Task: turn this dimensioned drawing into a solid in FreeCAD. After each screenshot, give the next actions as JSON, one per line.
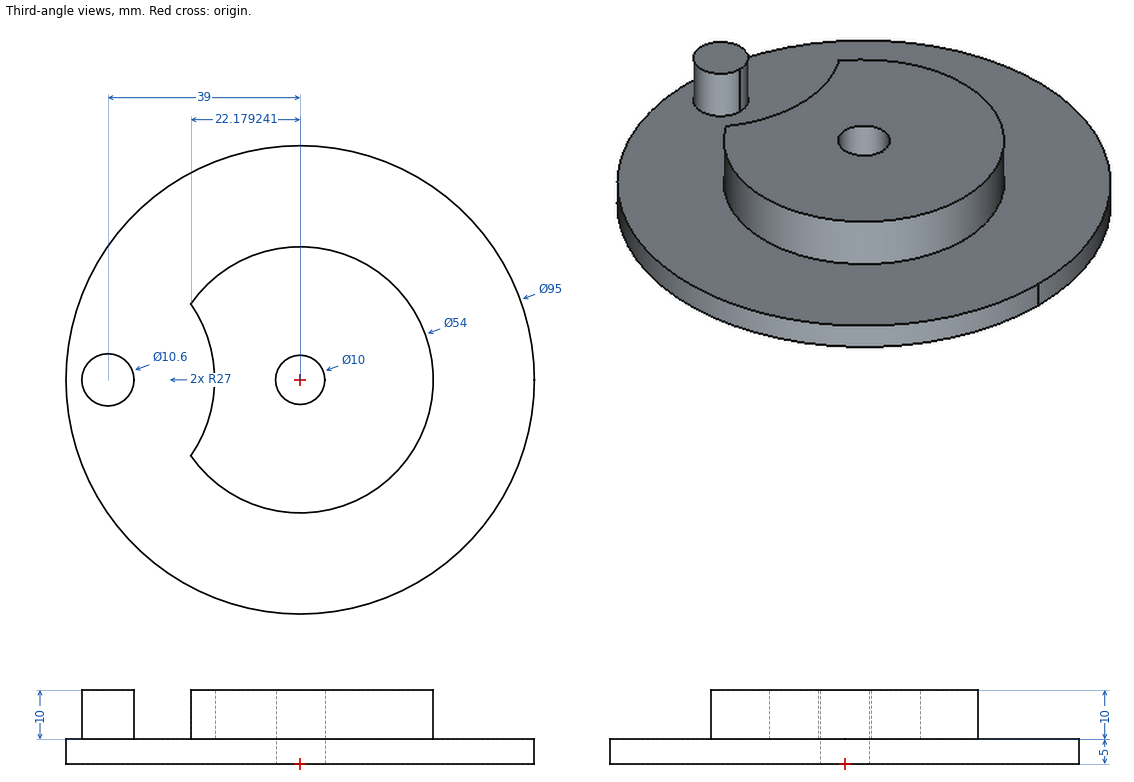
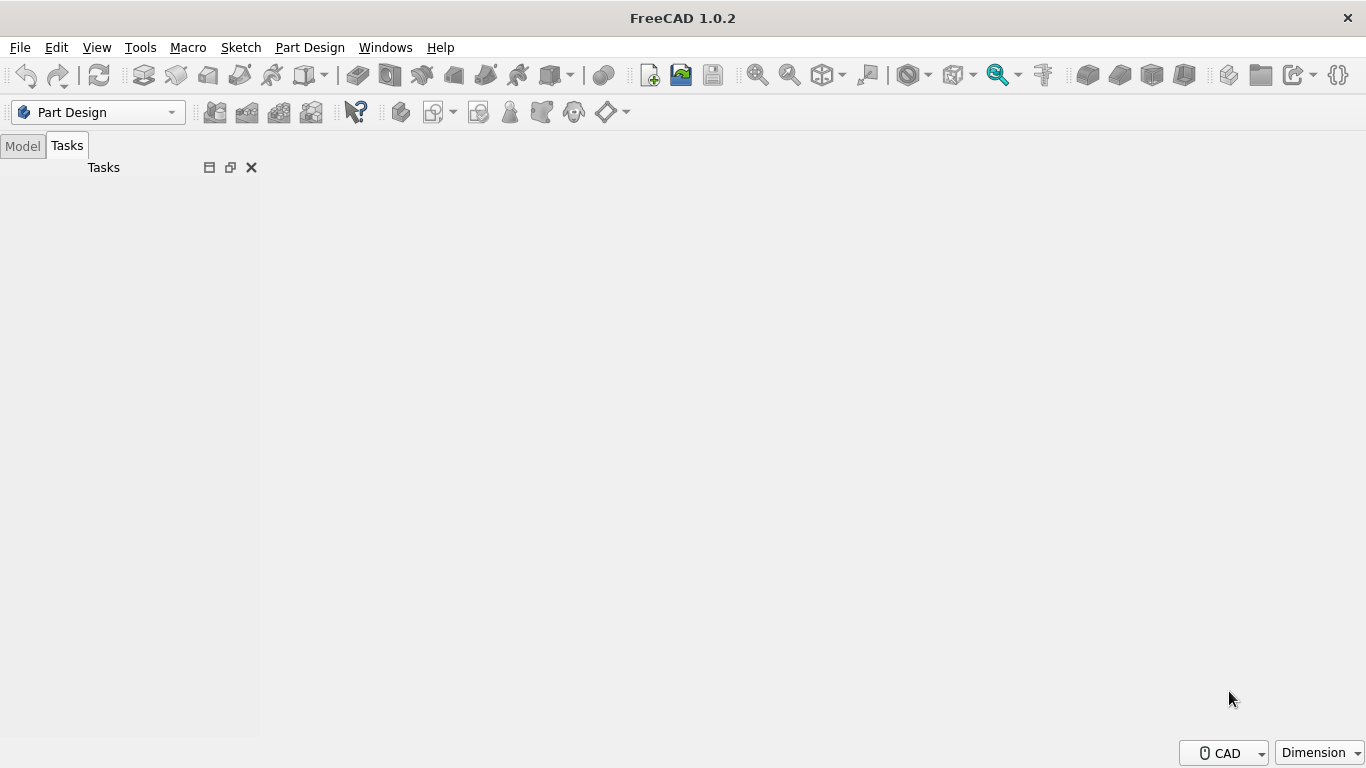
{"action": "key", "text": "ctrl+n"}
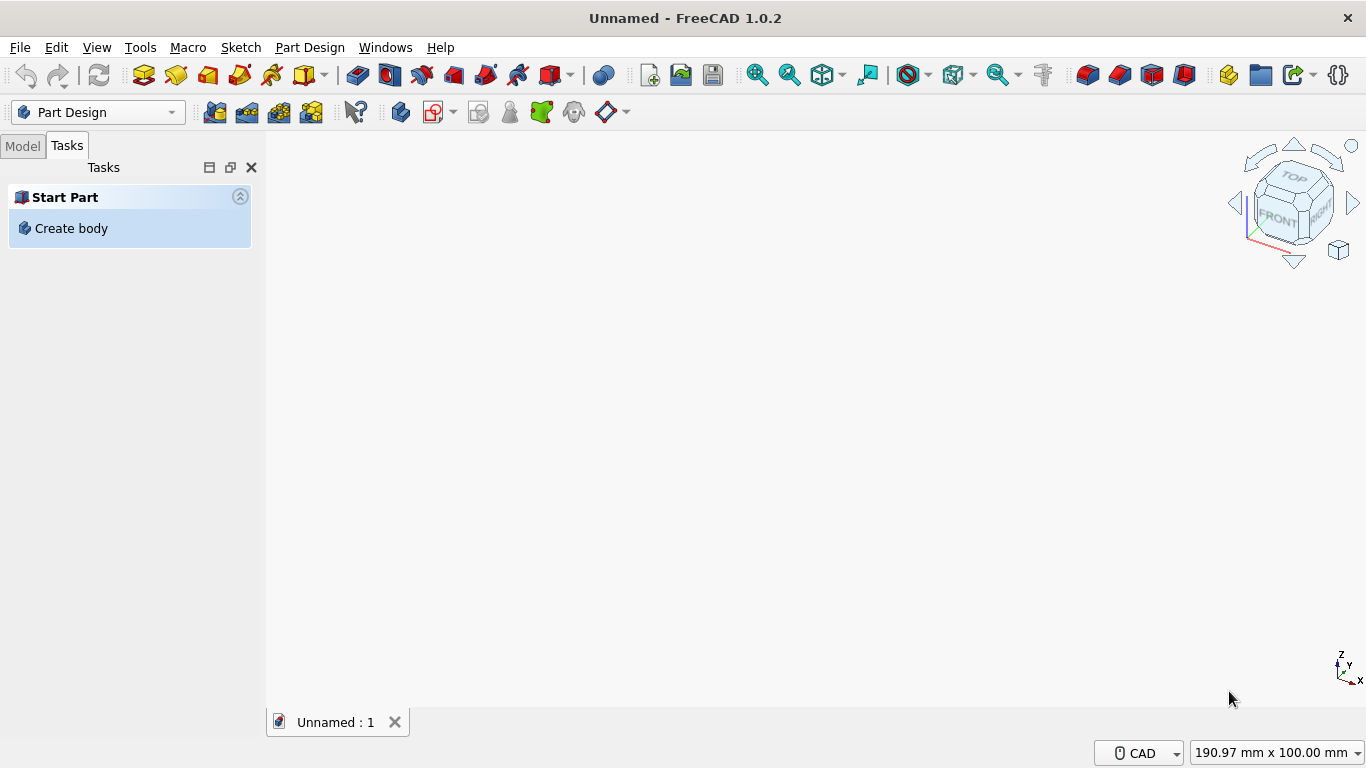
{"action": "left_click", "coordinate": [434, 112]}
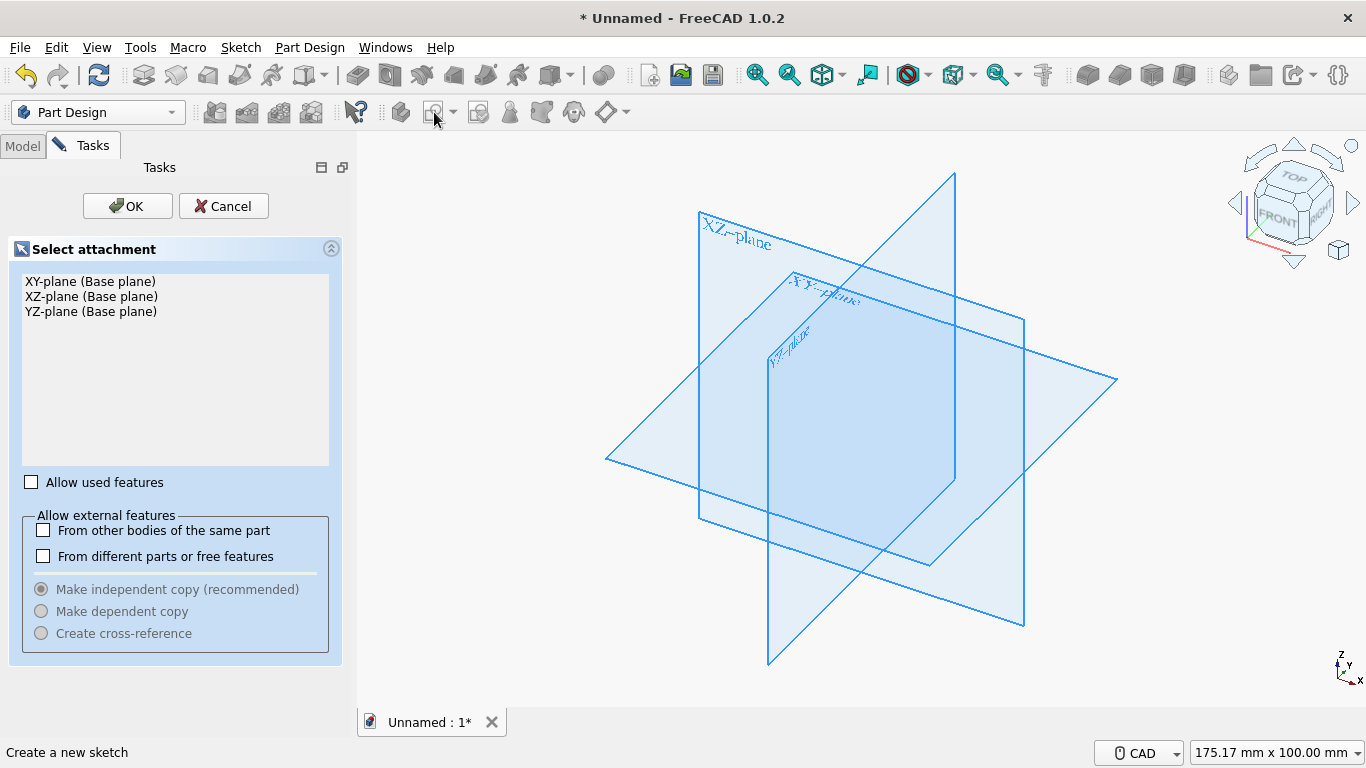
{"action": "left_click", "coordinate": [82, 282]}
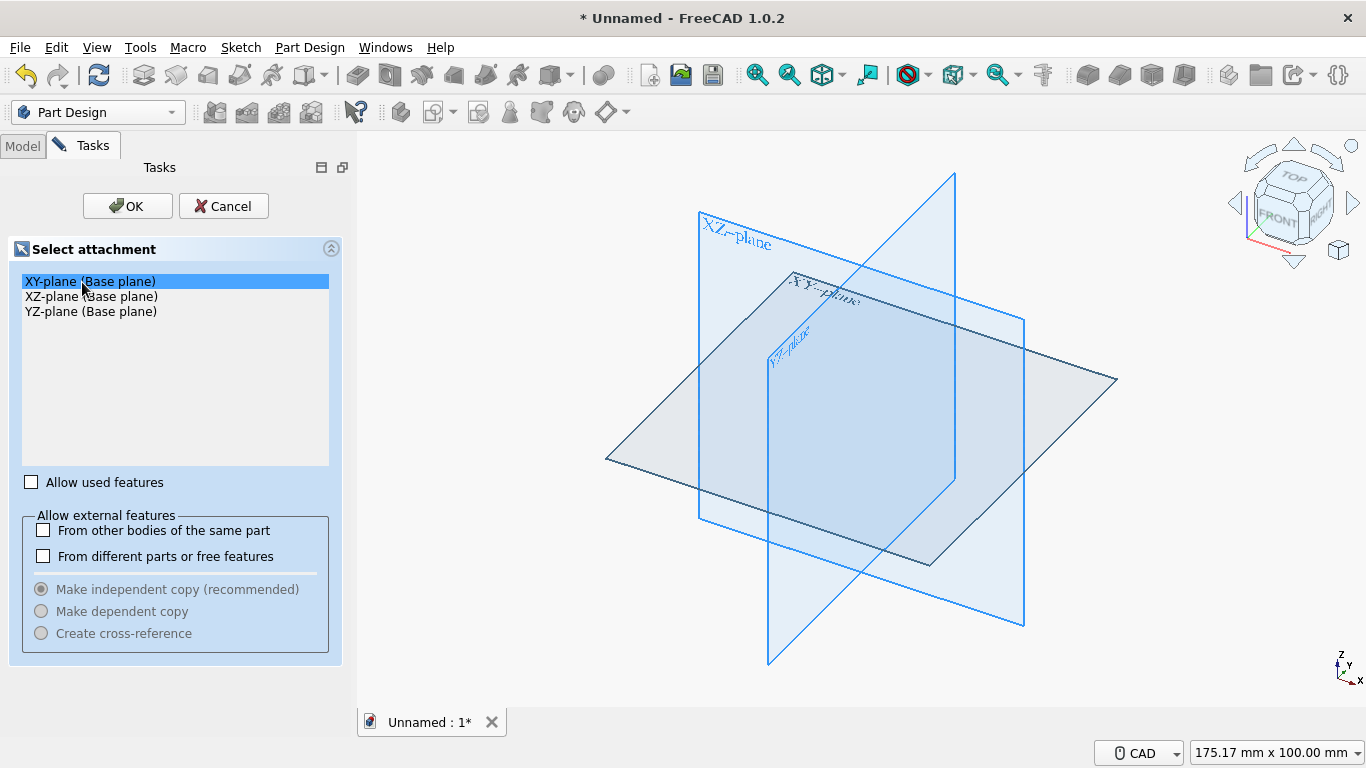
{"action": "left_click", "coordinate": [128, 206]}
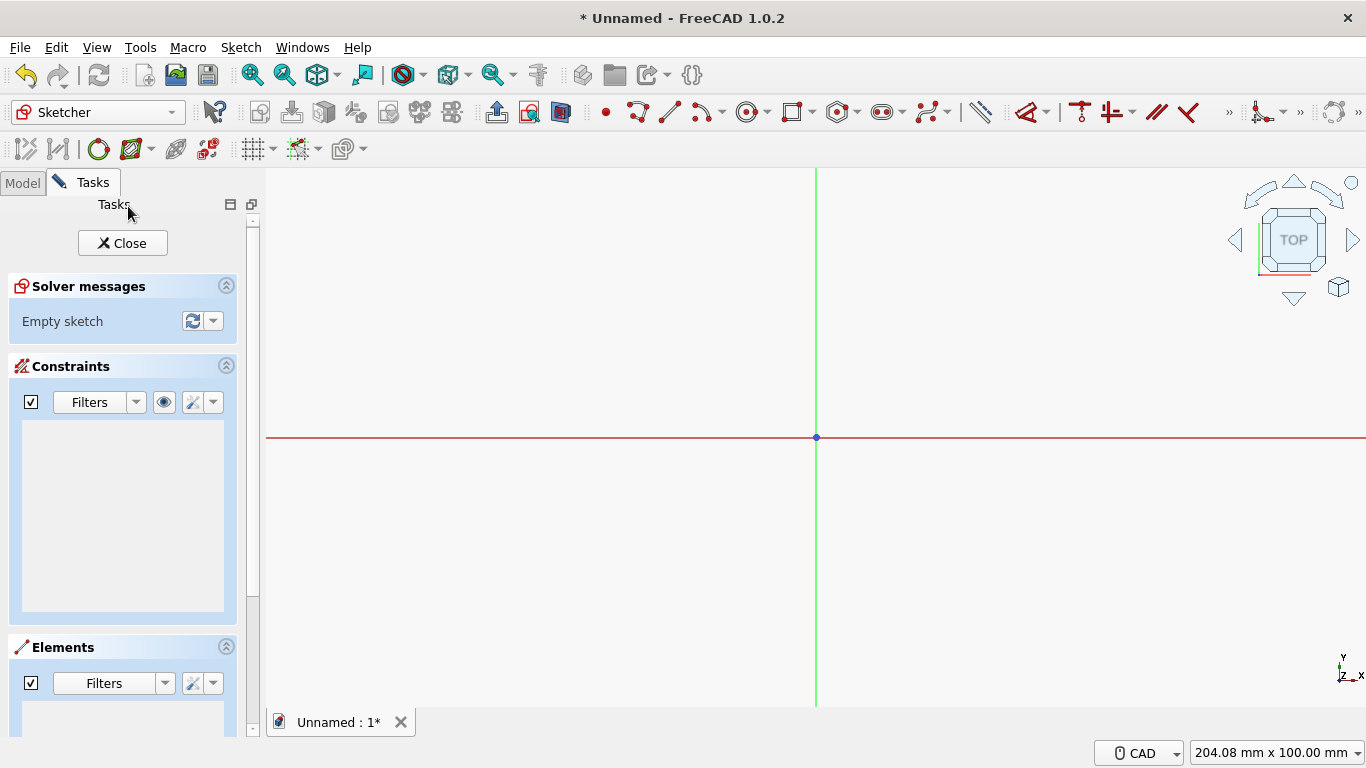
{"action": "scroll", "coordinate": [608, 438], "scroll_direction": "down", "scroll_amount": 2}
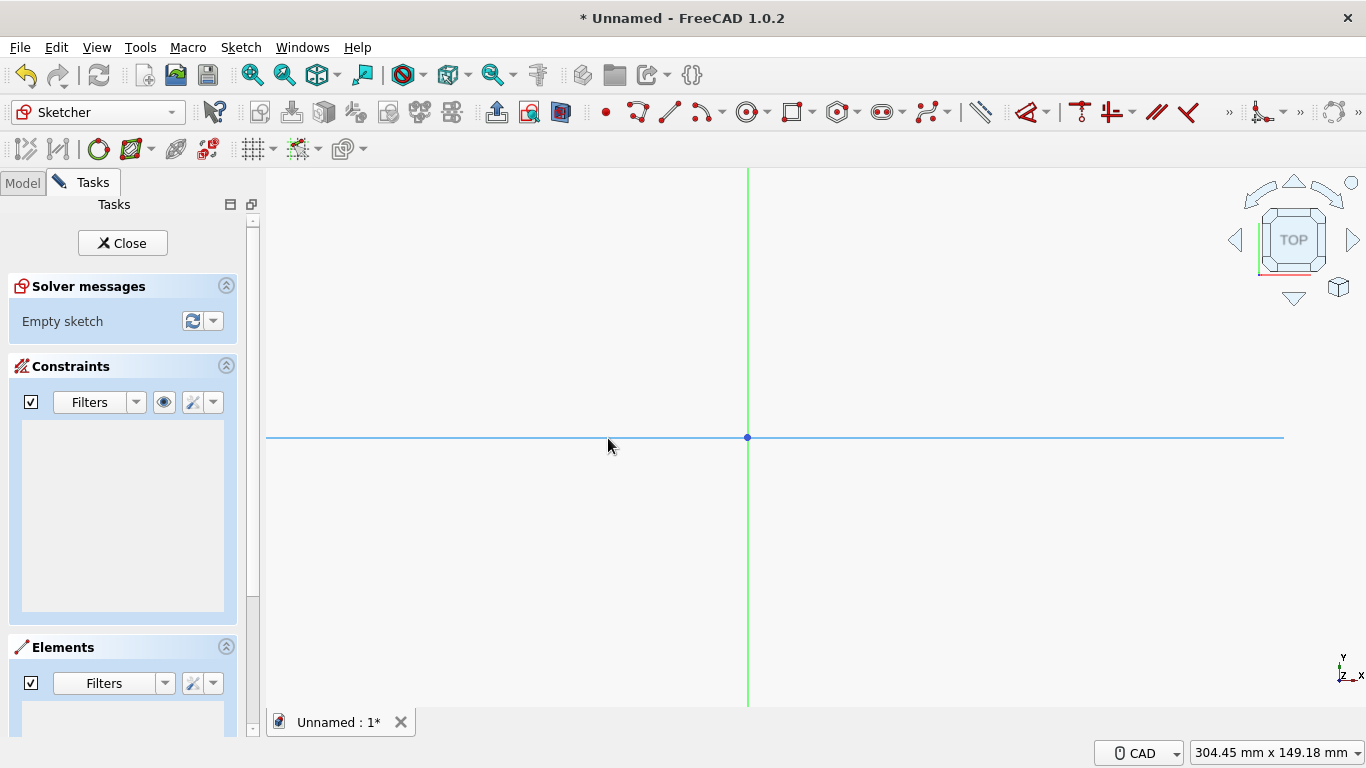
{"action": "key", "text": "g c"}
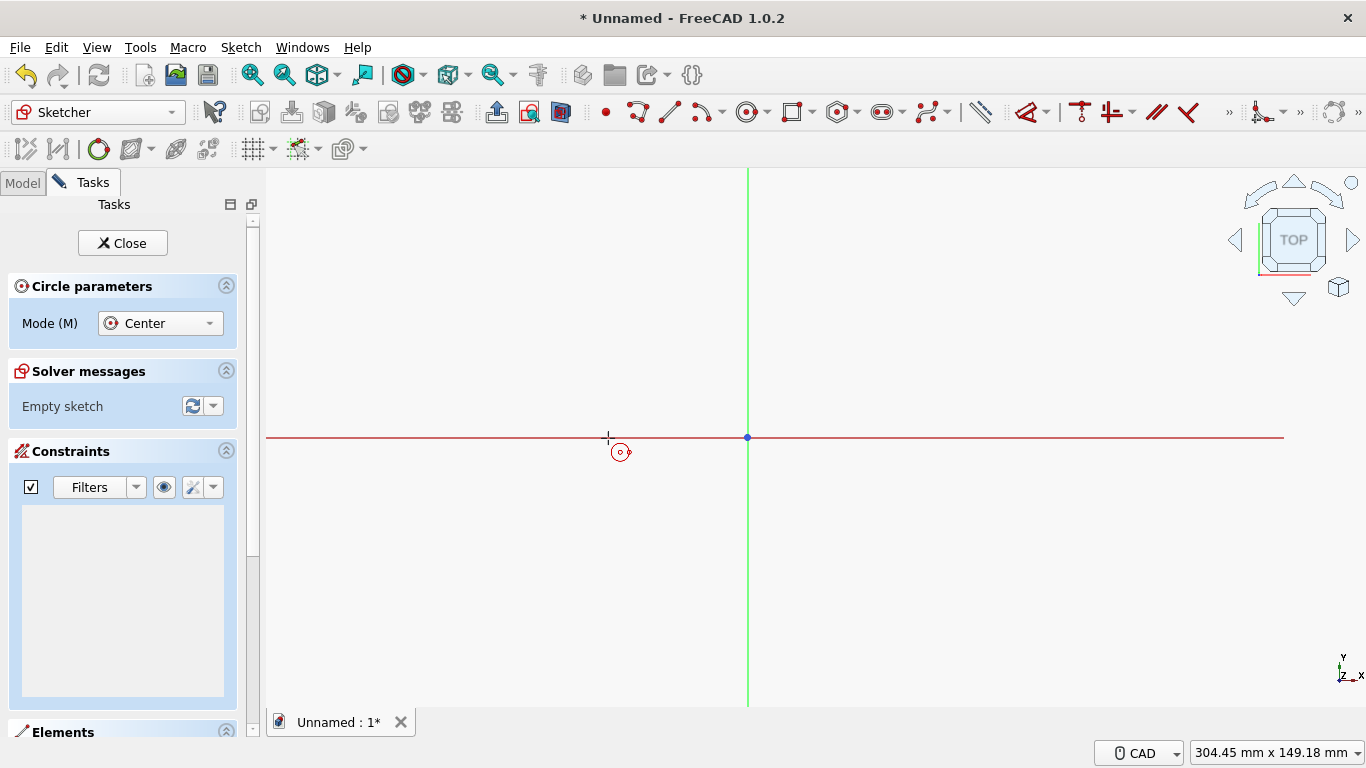
{"action": "left_click", "coordinate": [748, 438]}
{"action": "left_click", "coordinate": [869, 316]}
{"action": "key", "text": "Escape"}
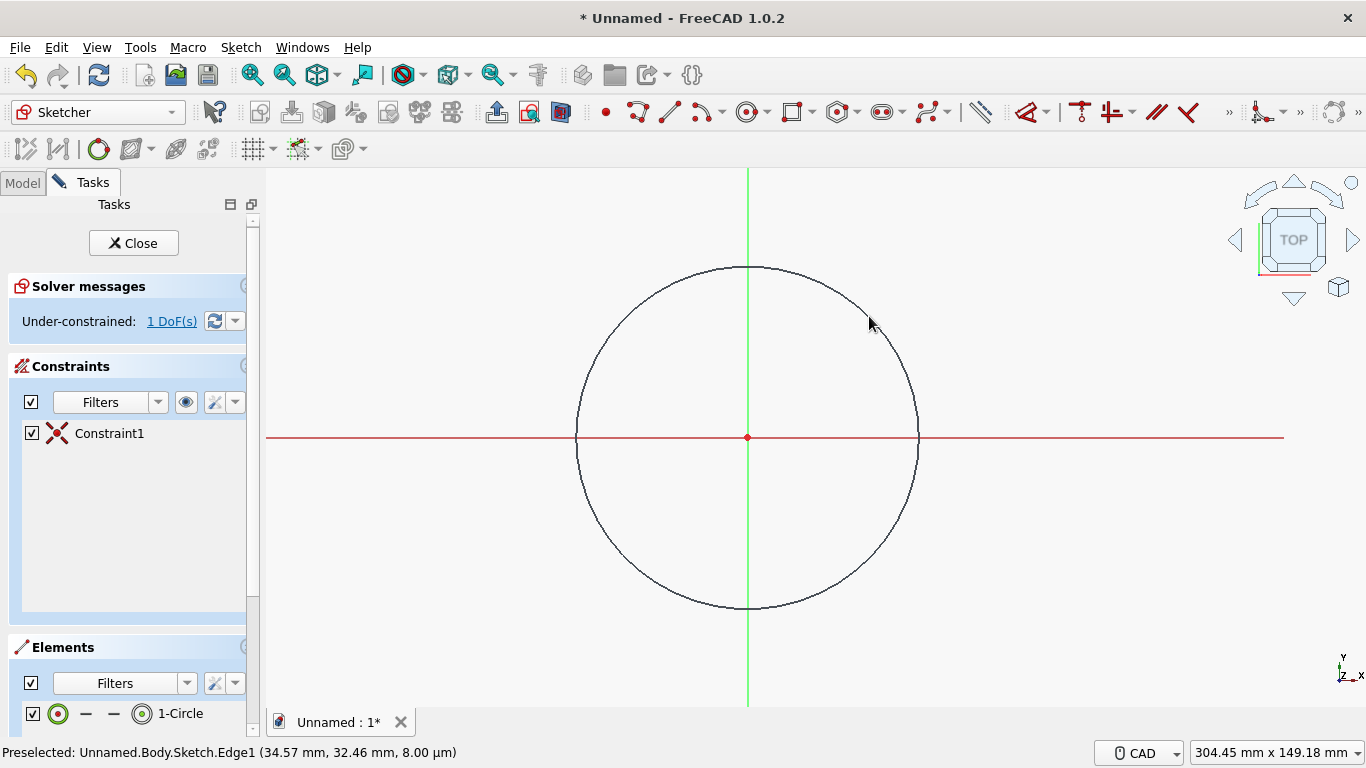
{"action": "key", "text": "d"}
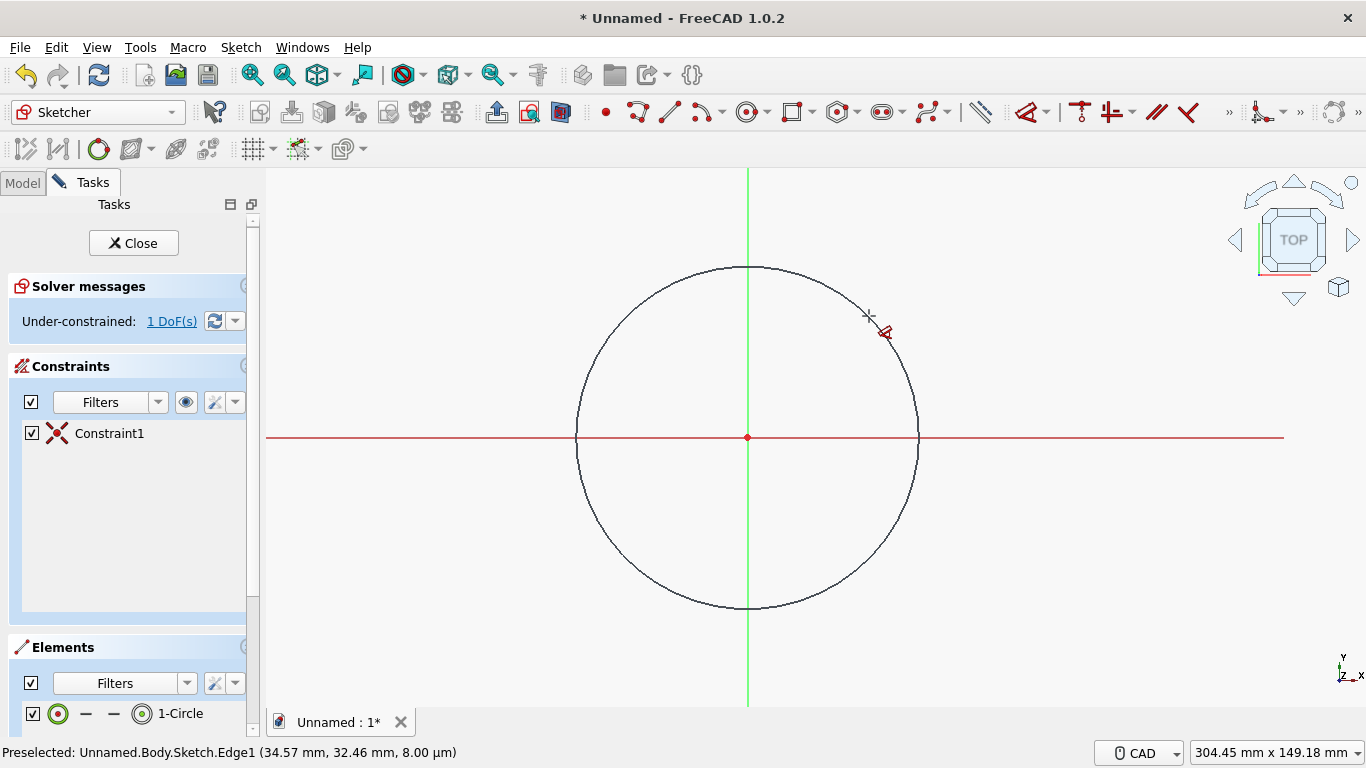
{"action": "left_click", "coordinate": [868, 316]}
{"action": "left_click", "coordinate": [891, 293]}